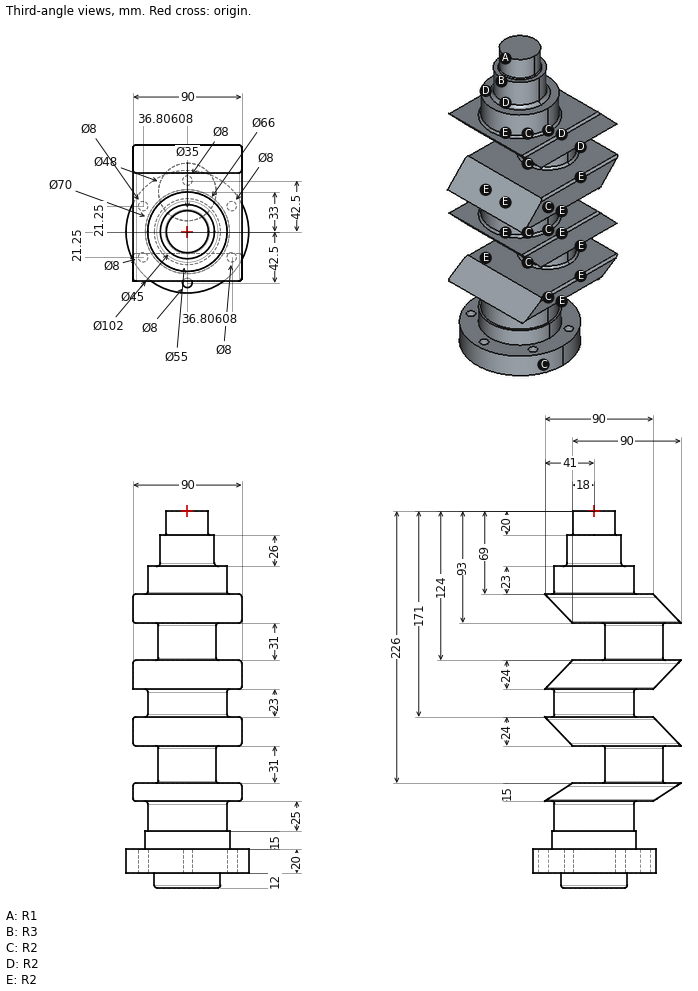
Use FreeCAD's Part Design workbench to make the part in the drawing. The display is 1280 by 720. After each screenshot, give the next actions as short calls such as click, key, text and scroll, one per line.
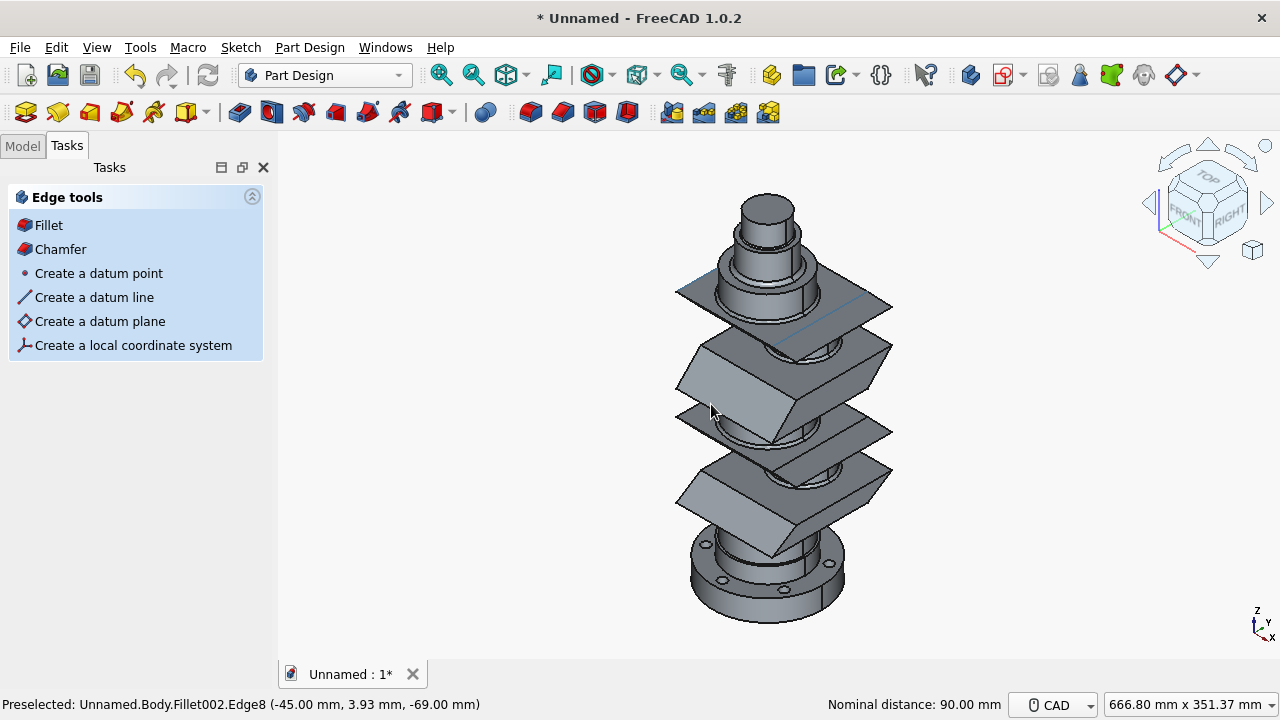
key(1)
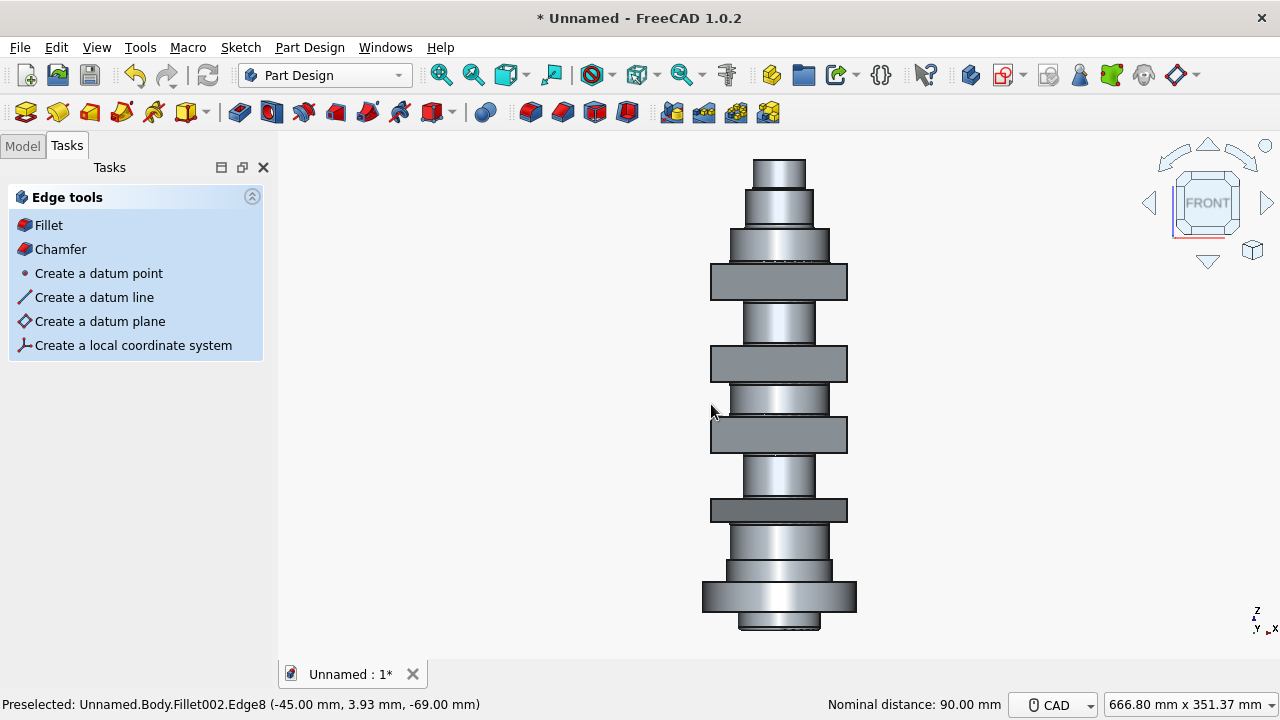
key(3)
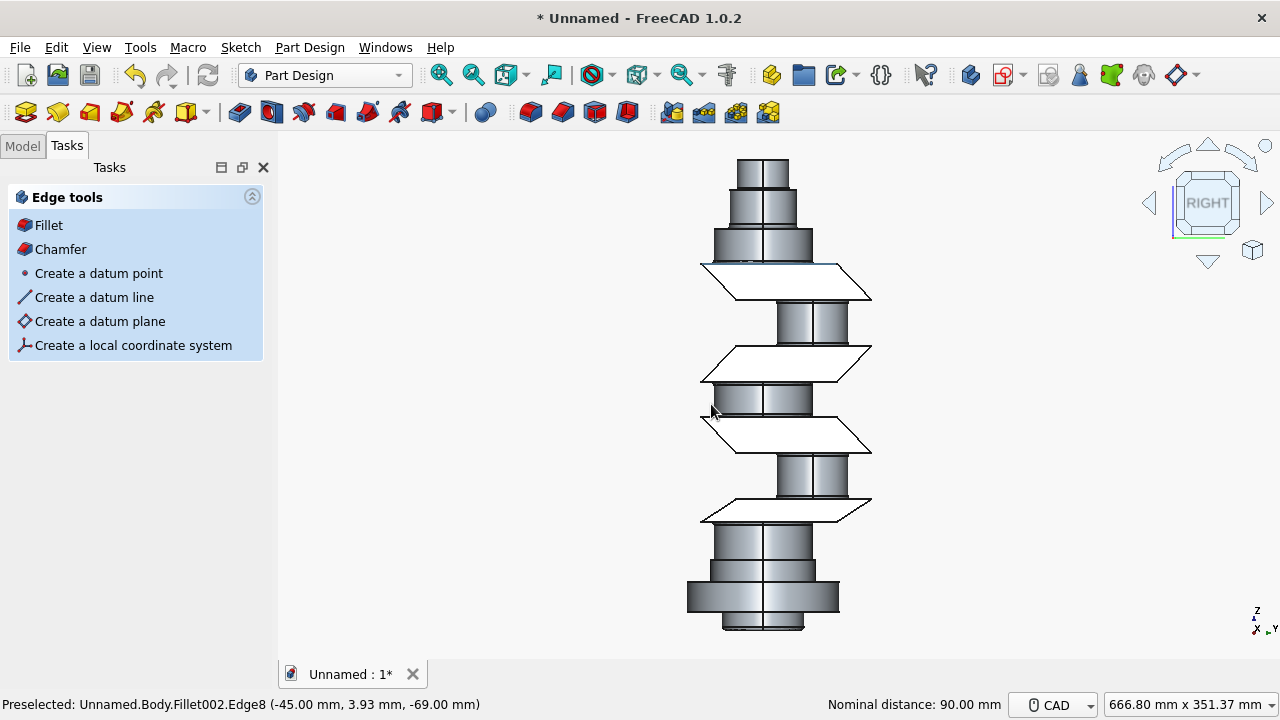
click(804, 299, ctrl)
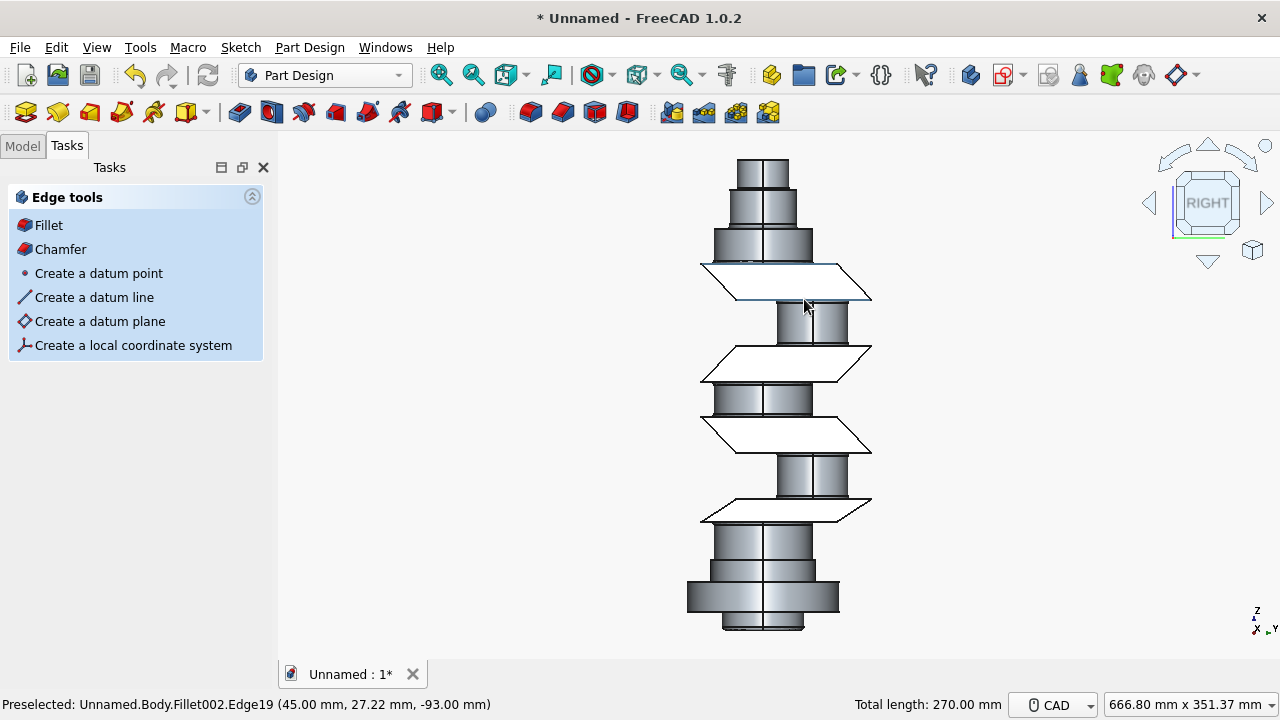
key(5)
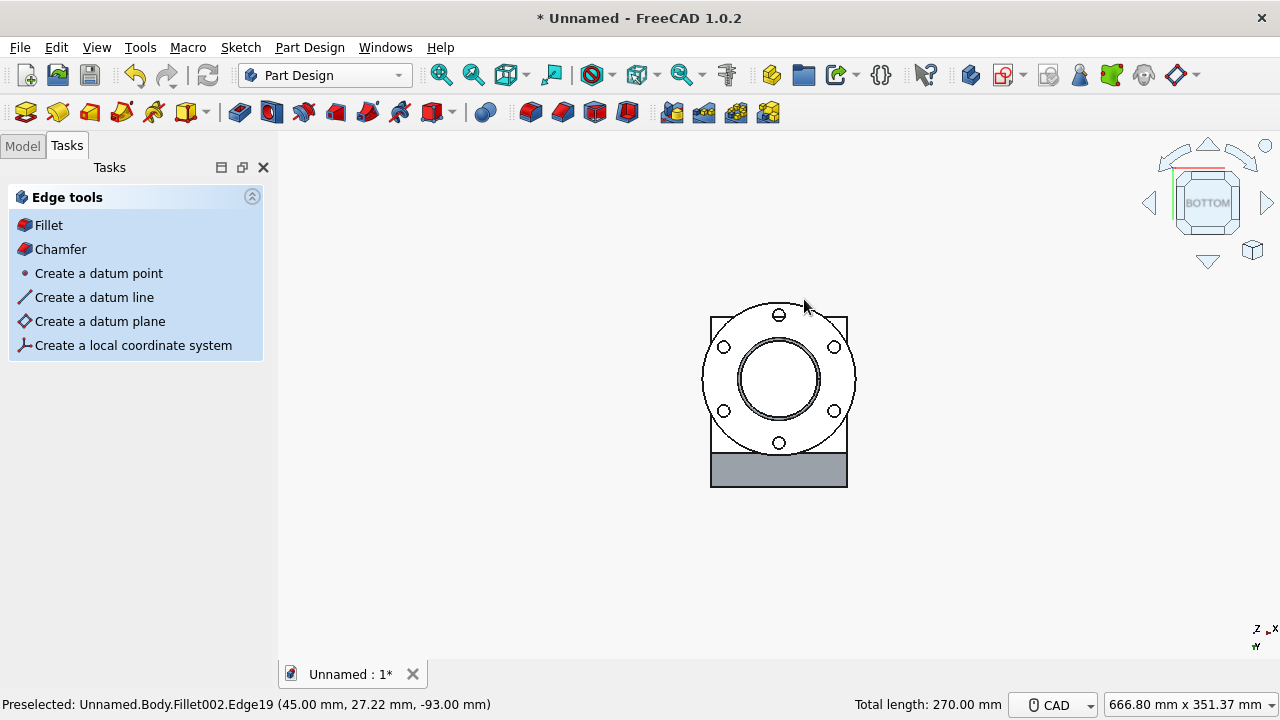
click(442, 76)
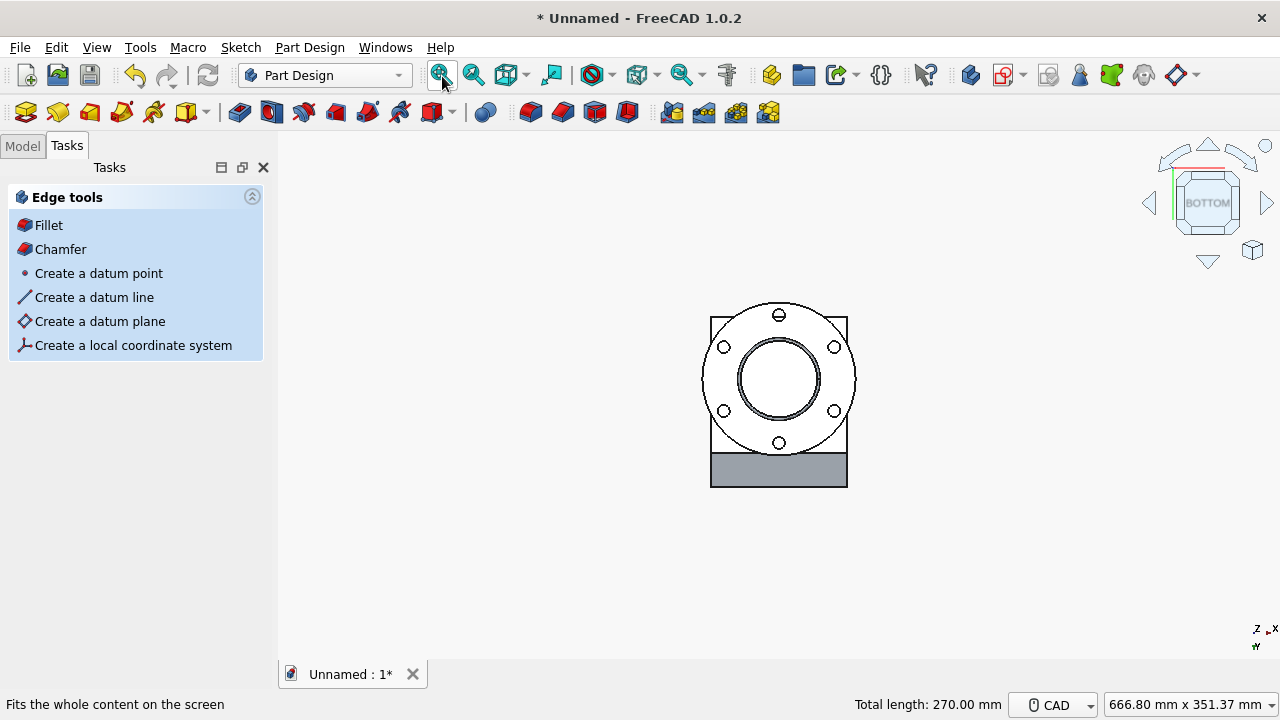
key(4)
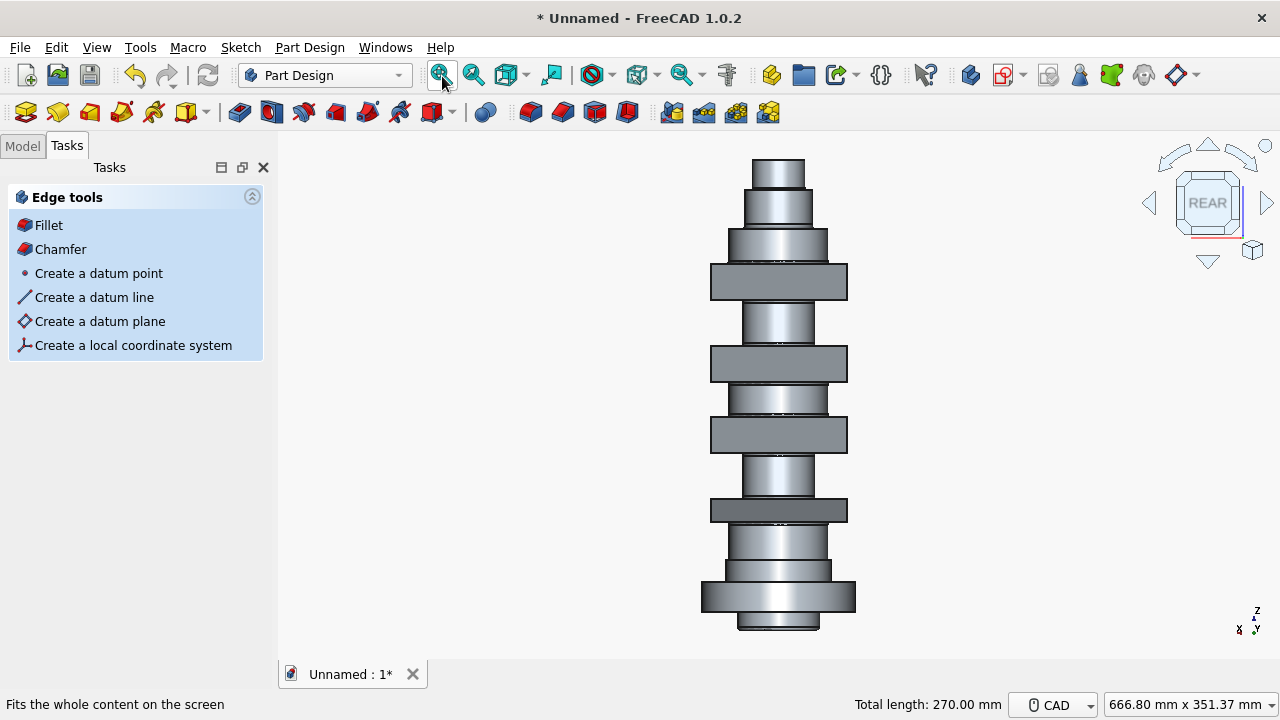
key(6)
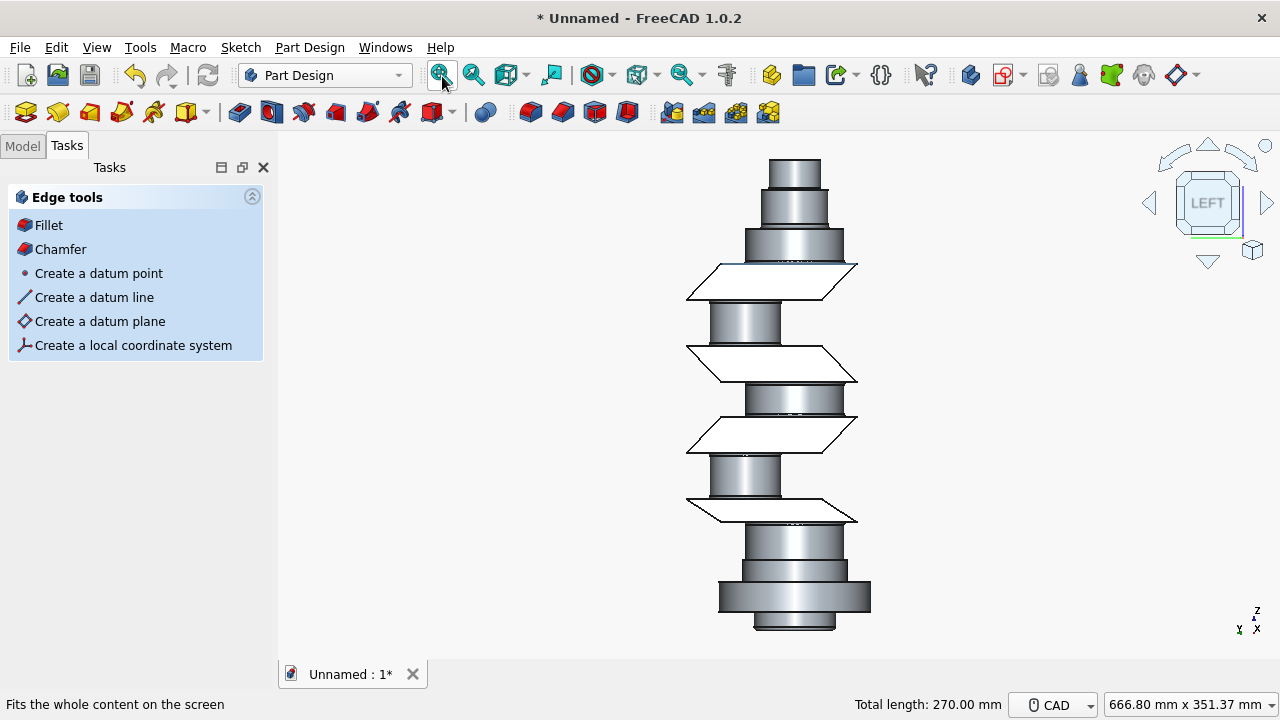
click(754, 299, ctrl)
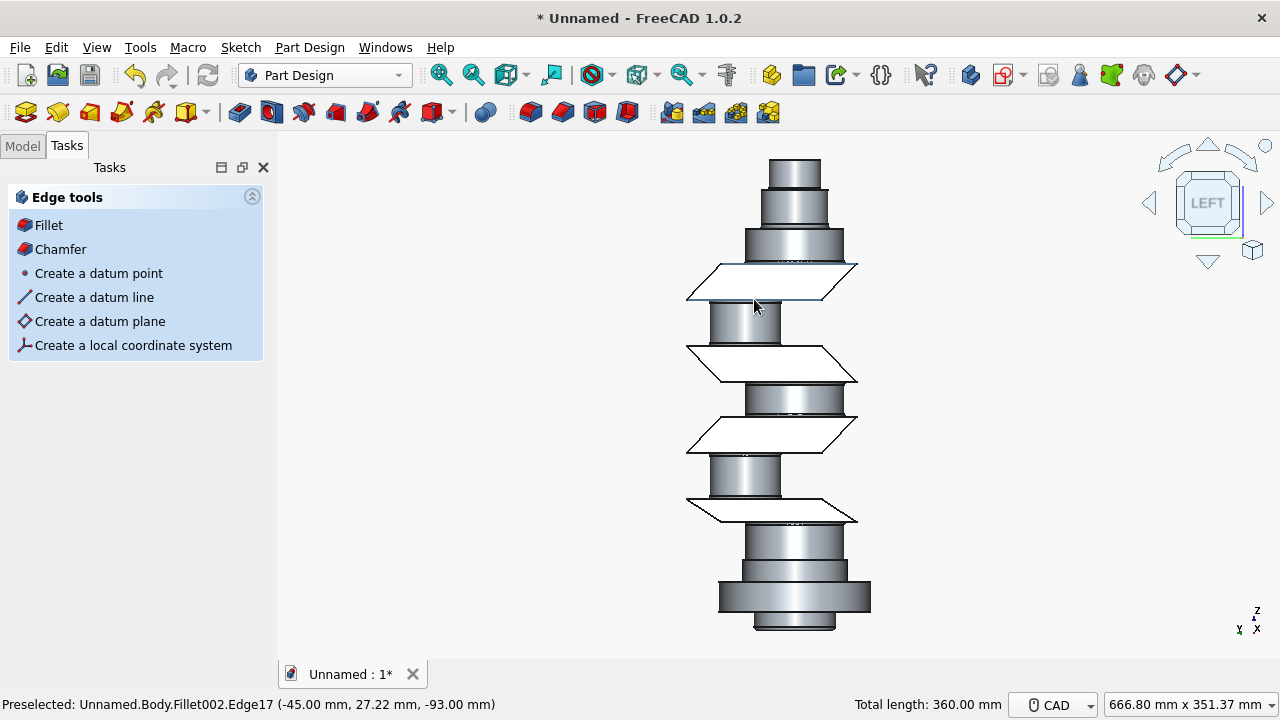
click(532, 112)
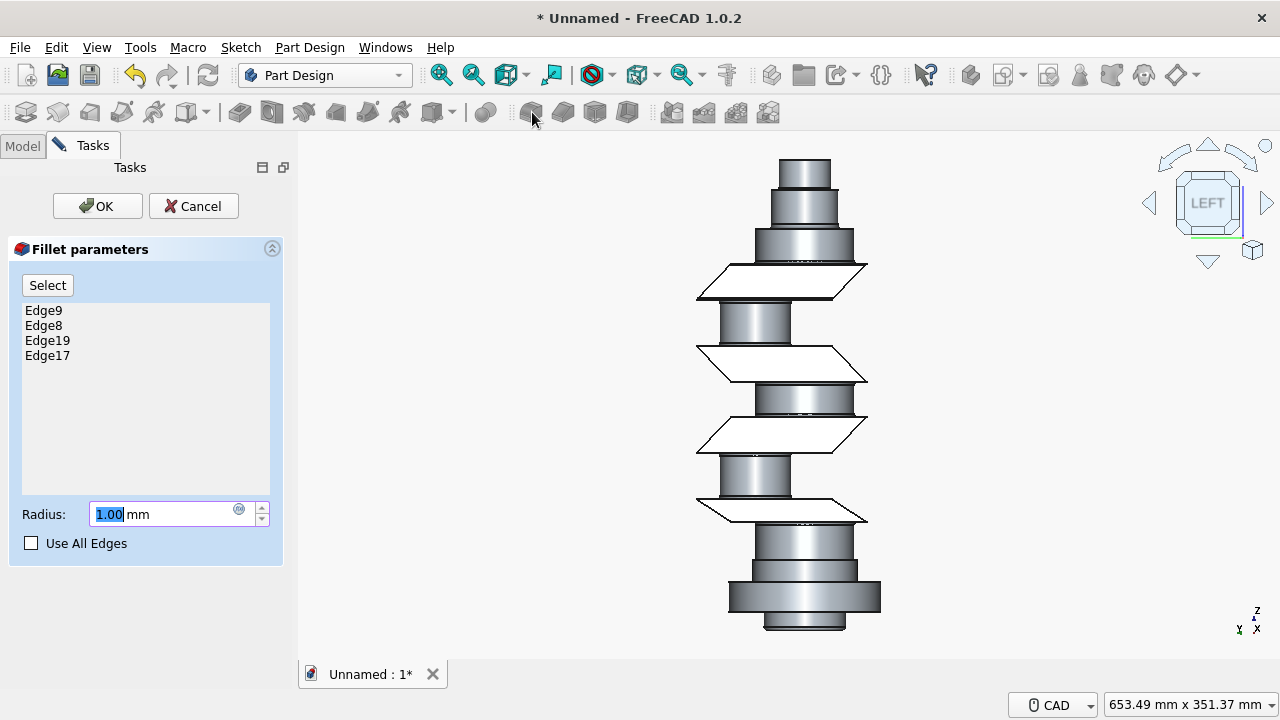
text(2)
key(Tab)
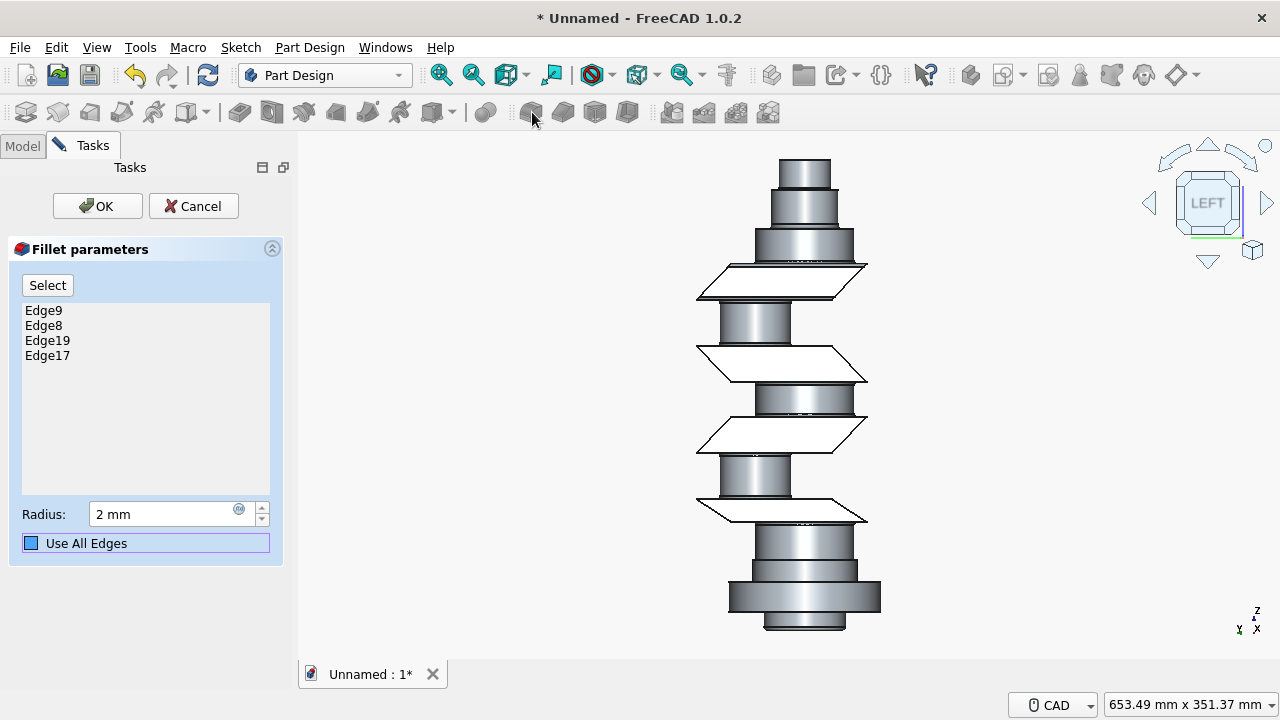
click(98, 206)